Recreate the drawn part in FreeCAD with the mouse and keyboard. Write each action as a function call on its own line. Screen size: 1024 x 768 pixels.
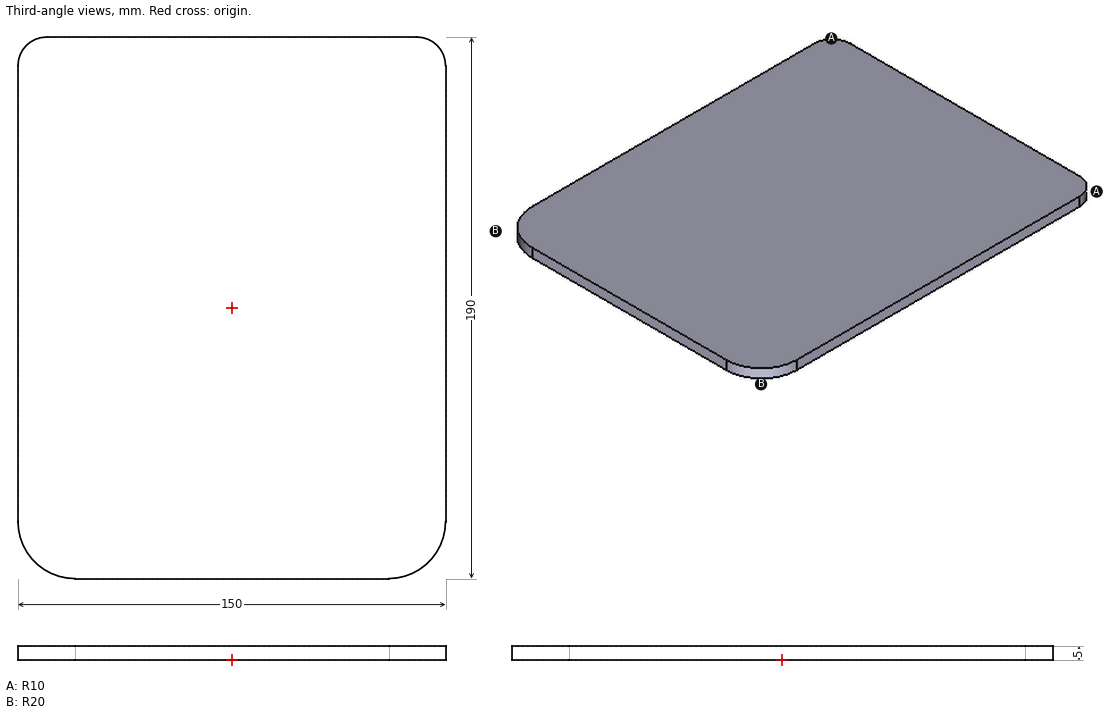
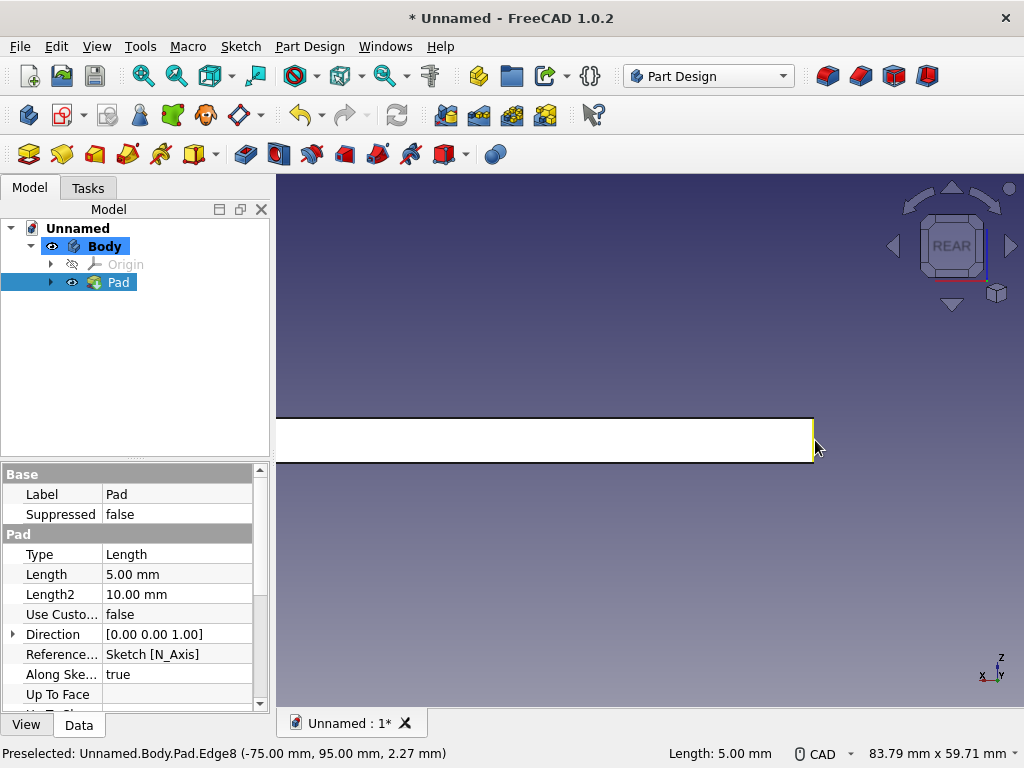
click(813, 440, ctrl)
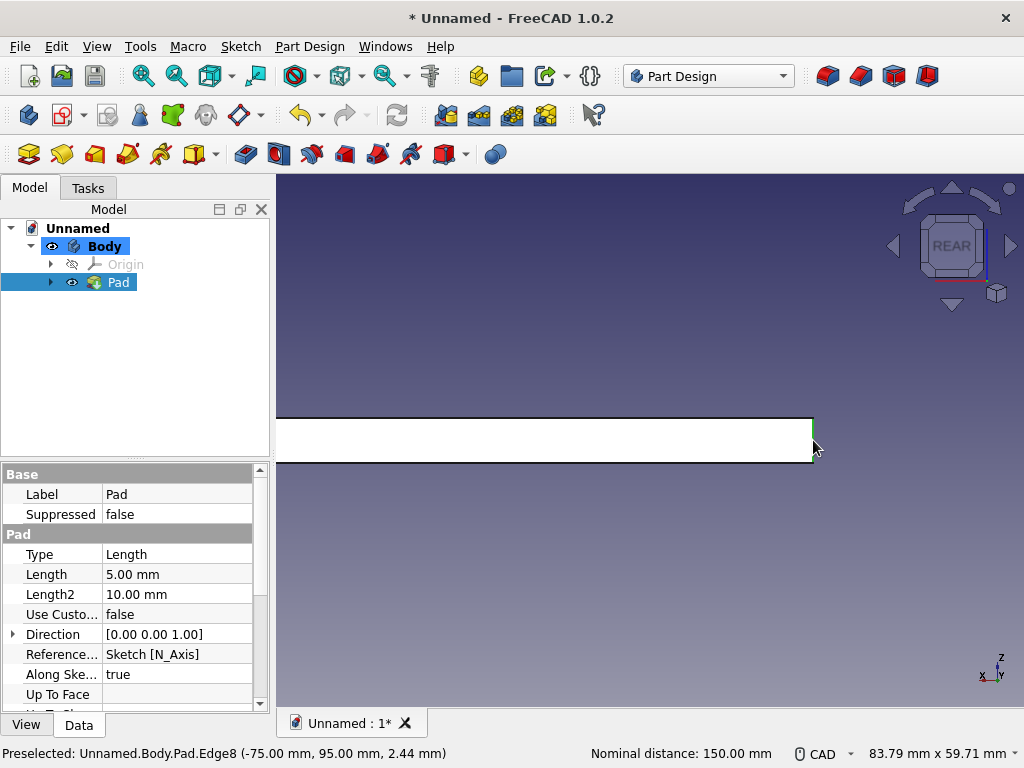
click(828, 76)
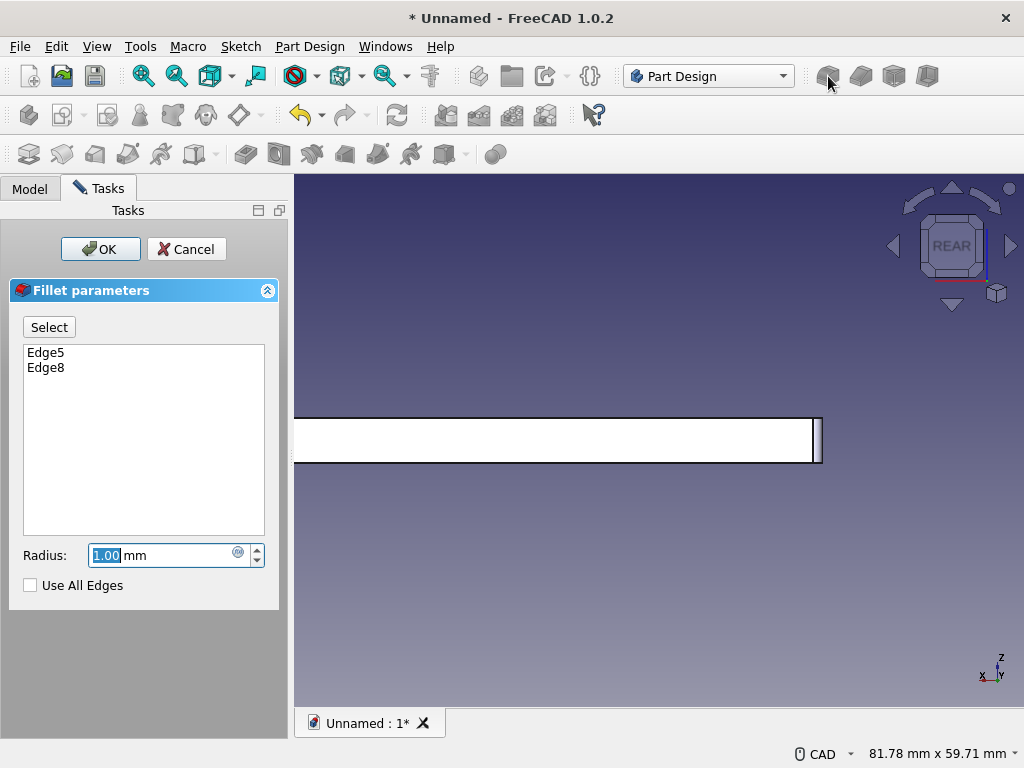
text(10)
key(Tab)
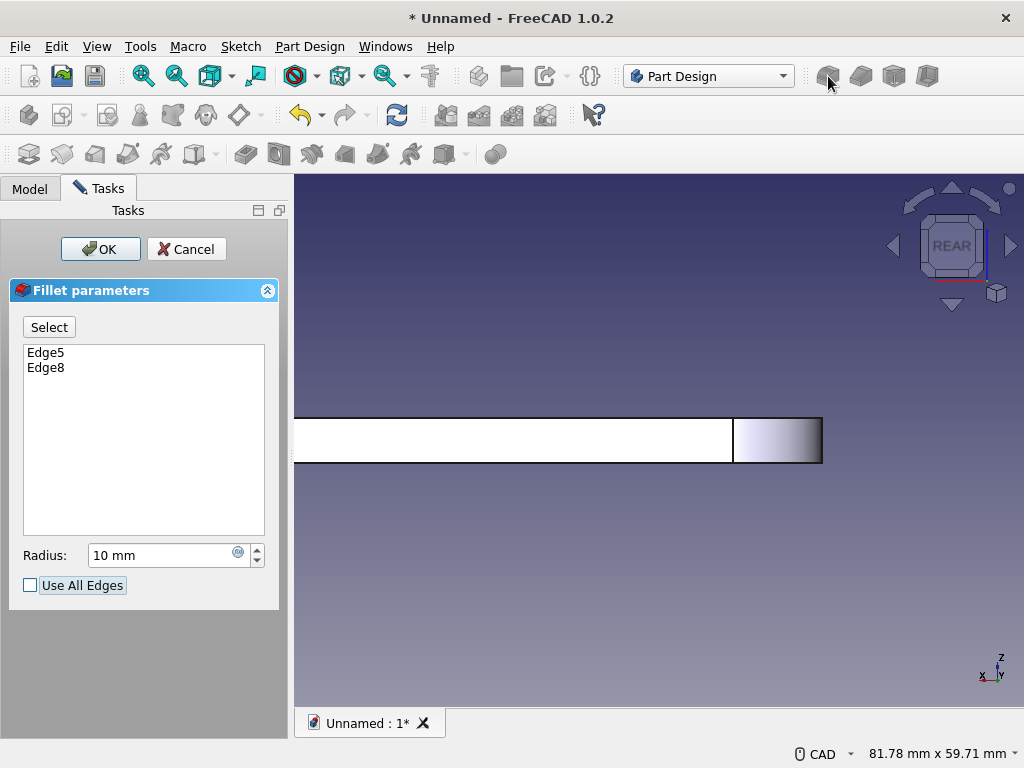
click(101, 249)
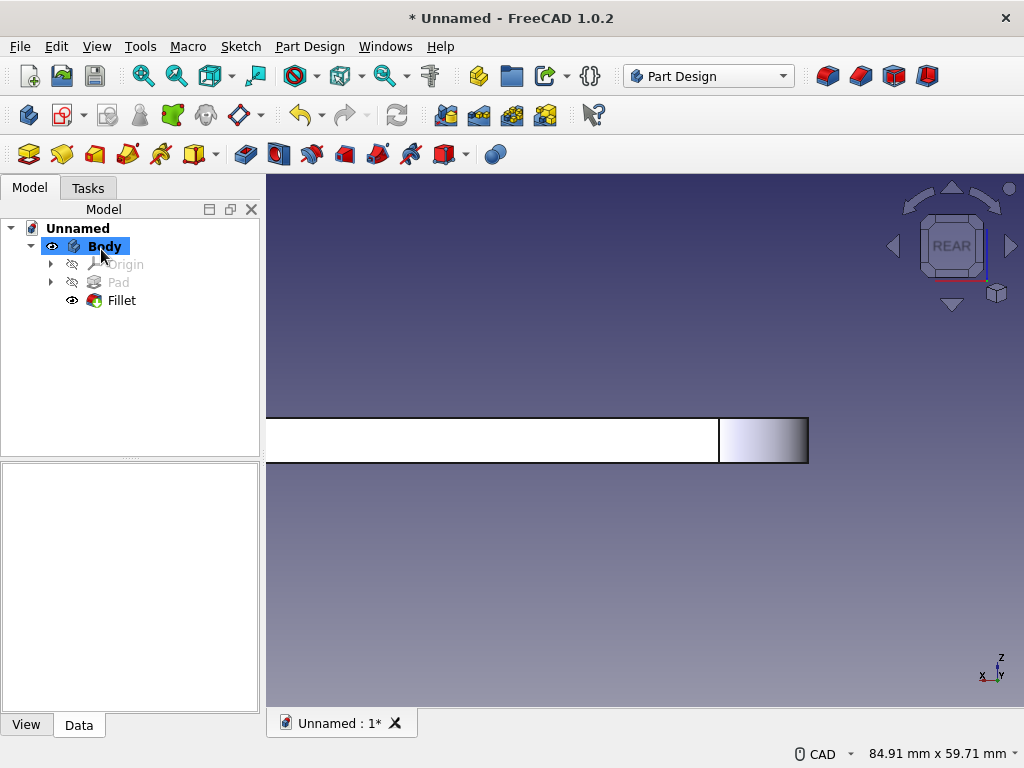
click(144, 76)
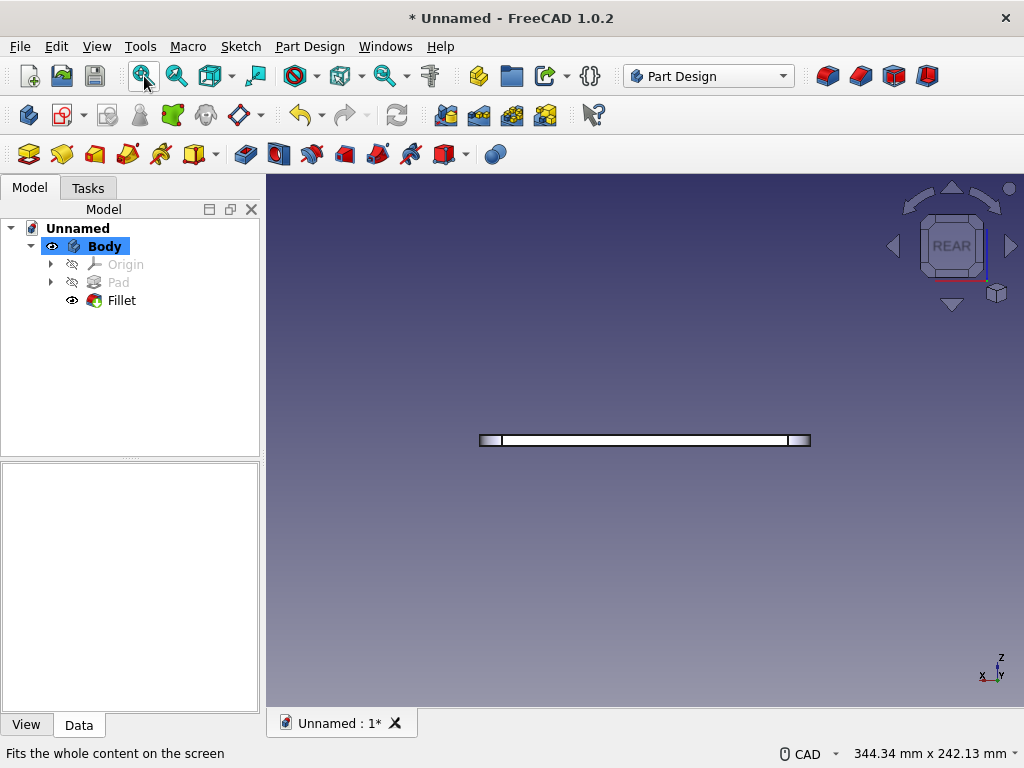
scroll(480, 440, up, 7)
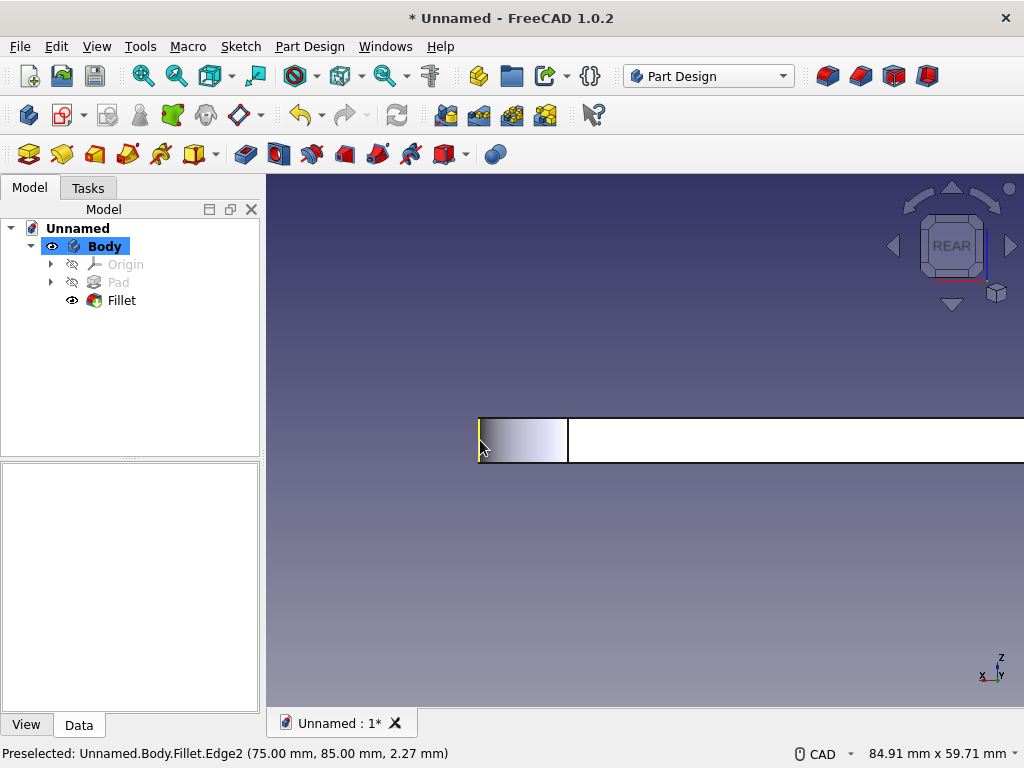
click(144, 76)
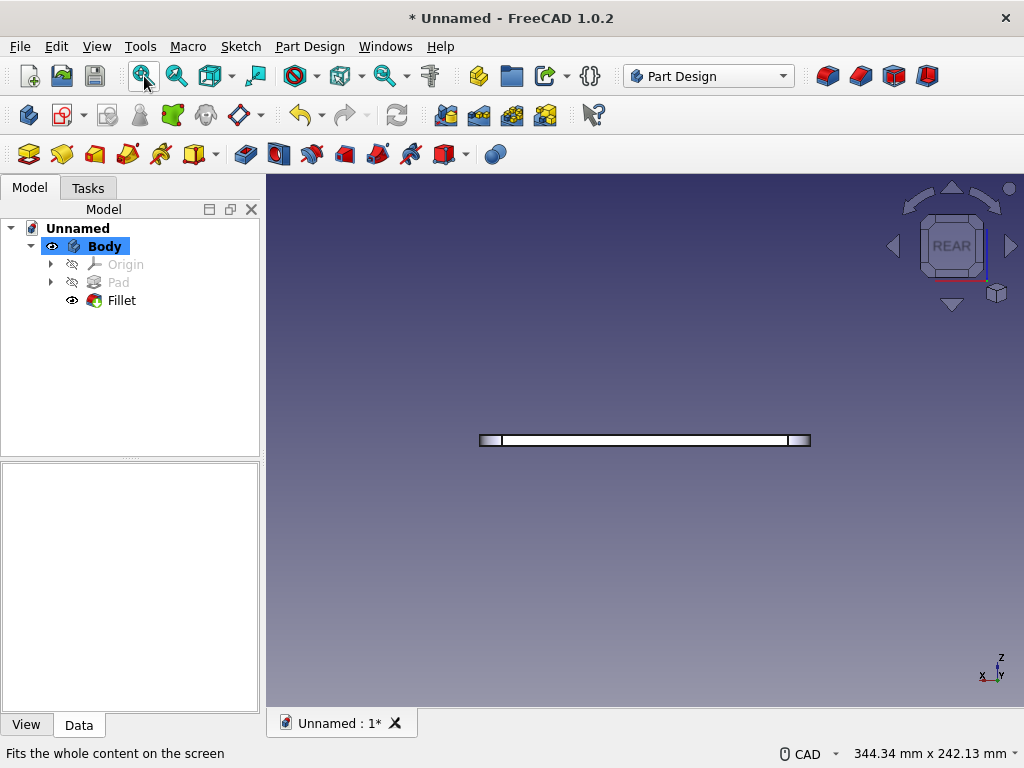
key(0)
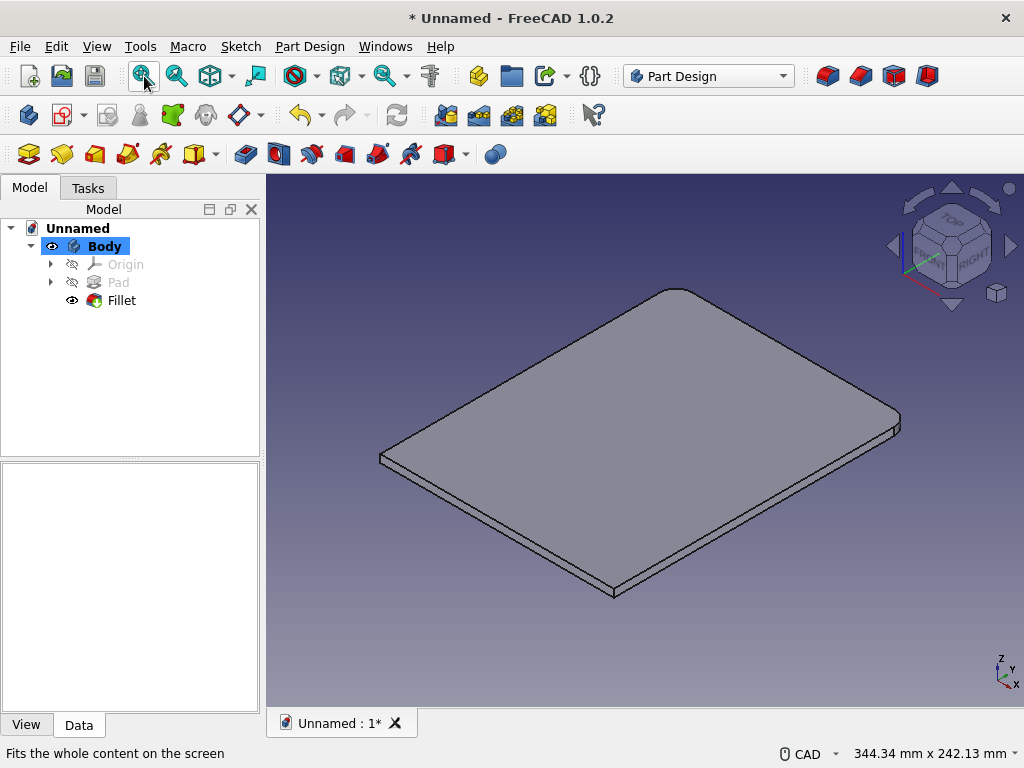
click(614, 594)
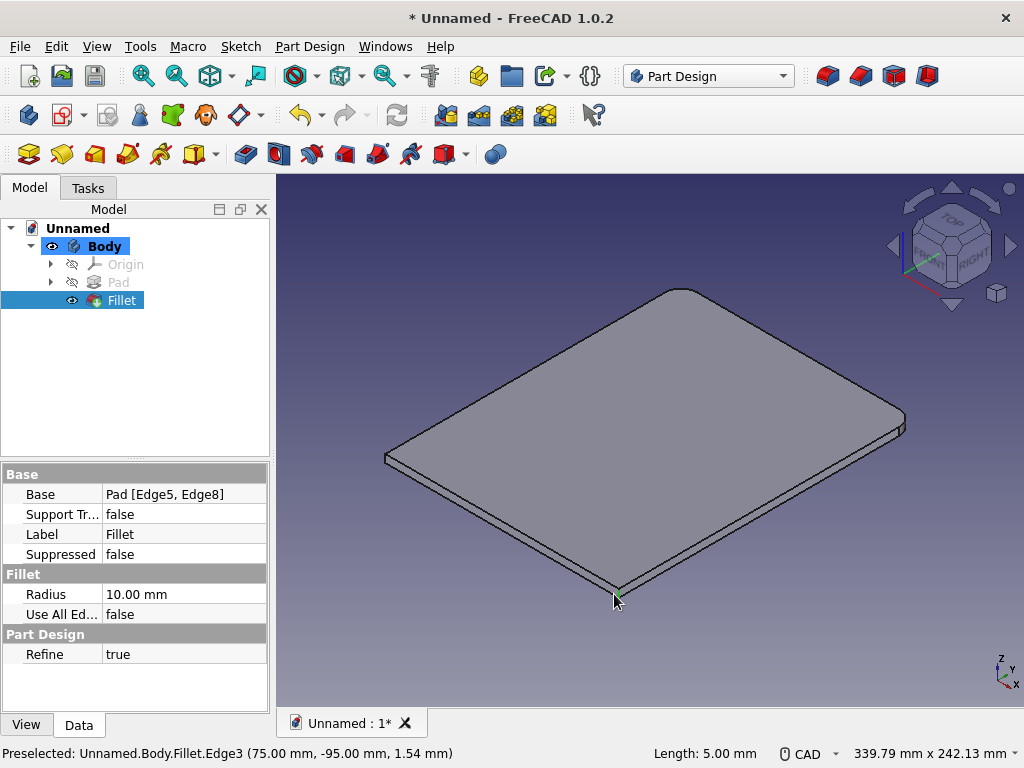
scroll(385, 457, up, 7)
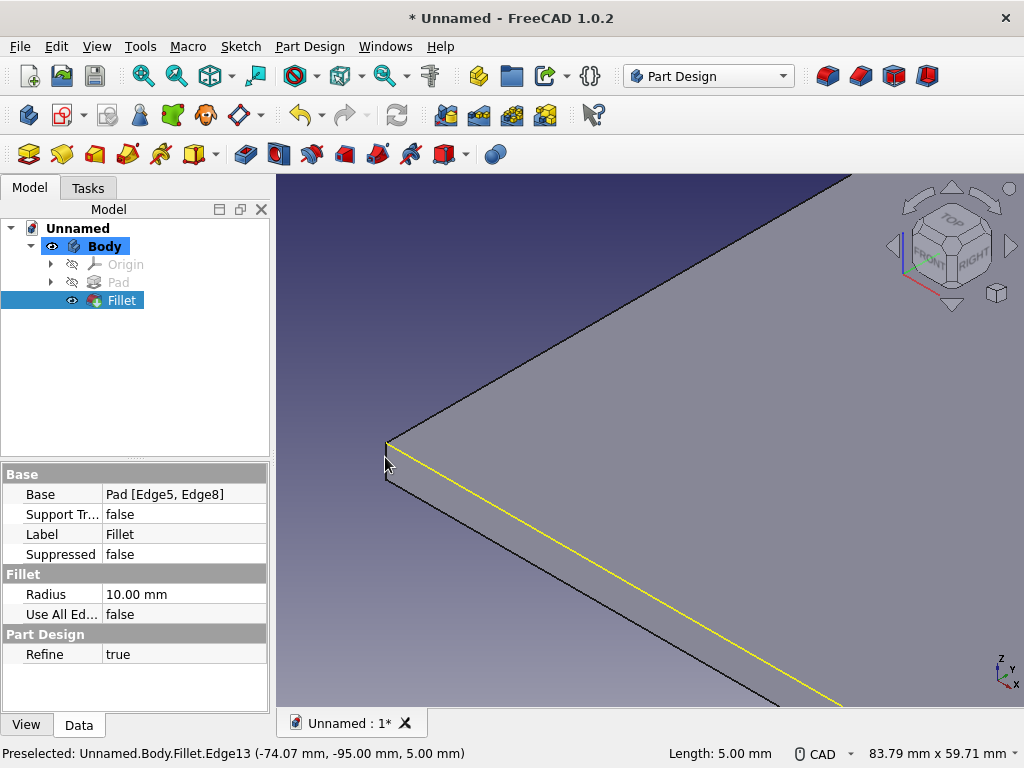
click(144, 76)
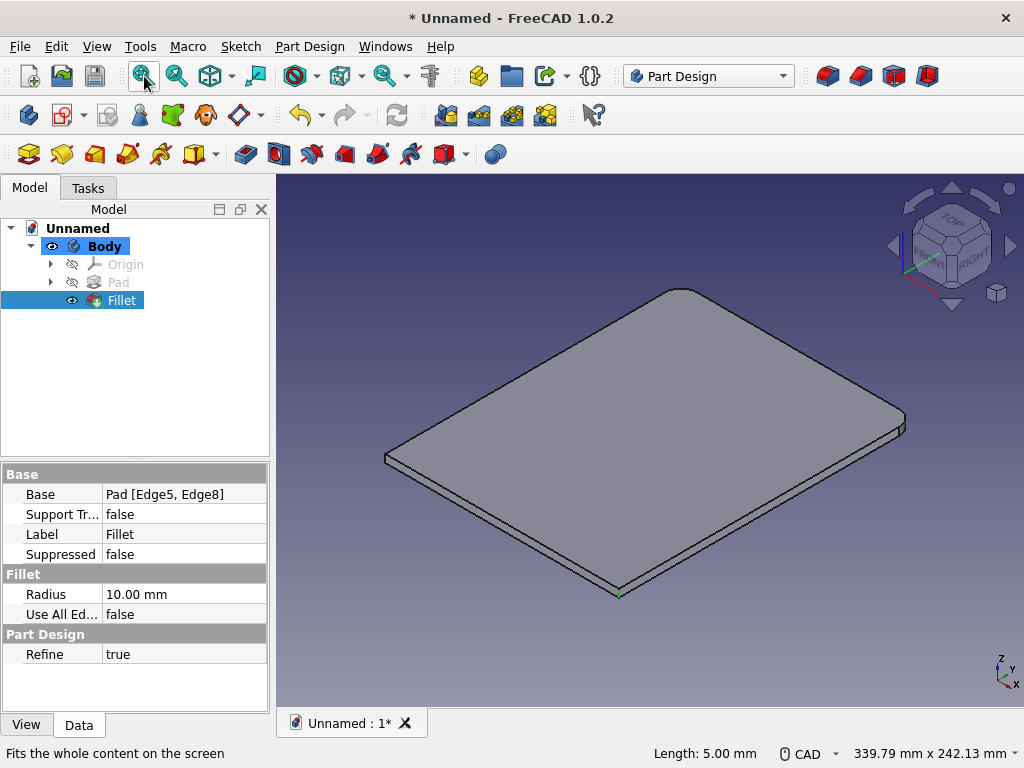
key(2)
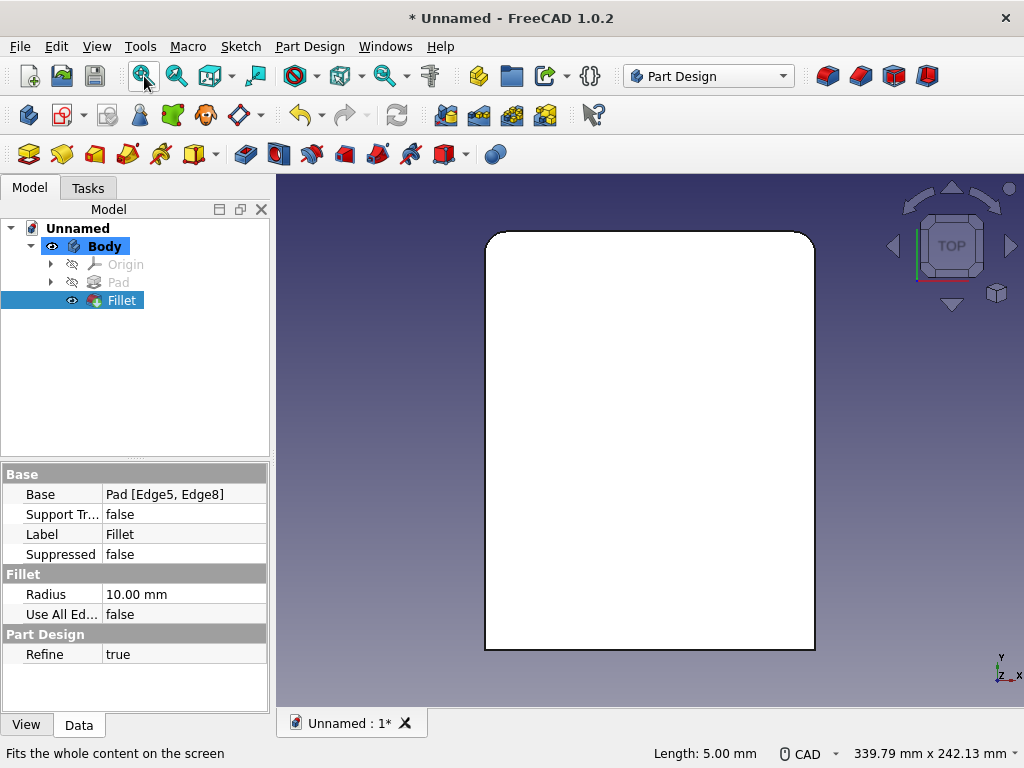
scroll(485, 649, up, 7)